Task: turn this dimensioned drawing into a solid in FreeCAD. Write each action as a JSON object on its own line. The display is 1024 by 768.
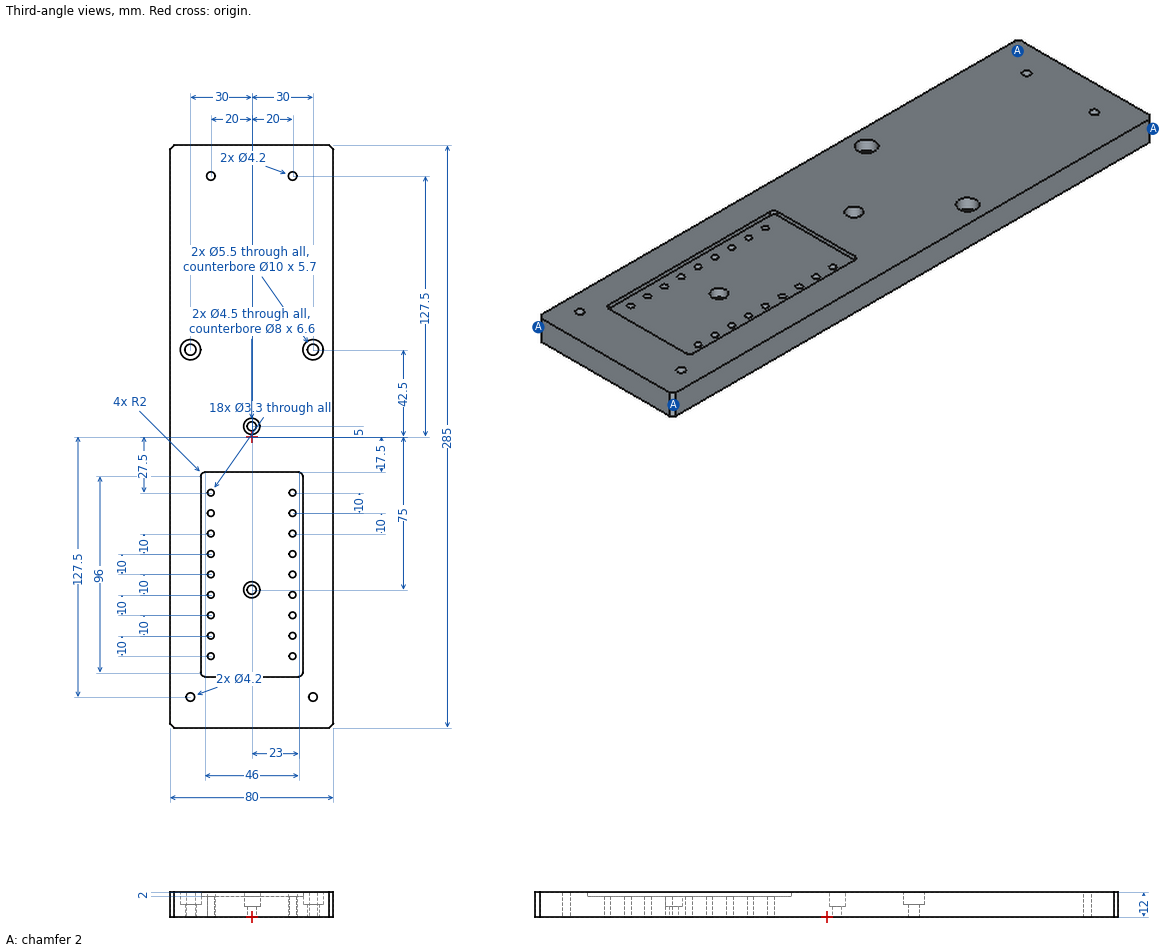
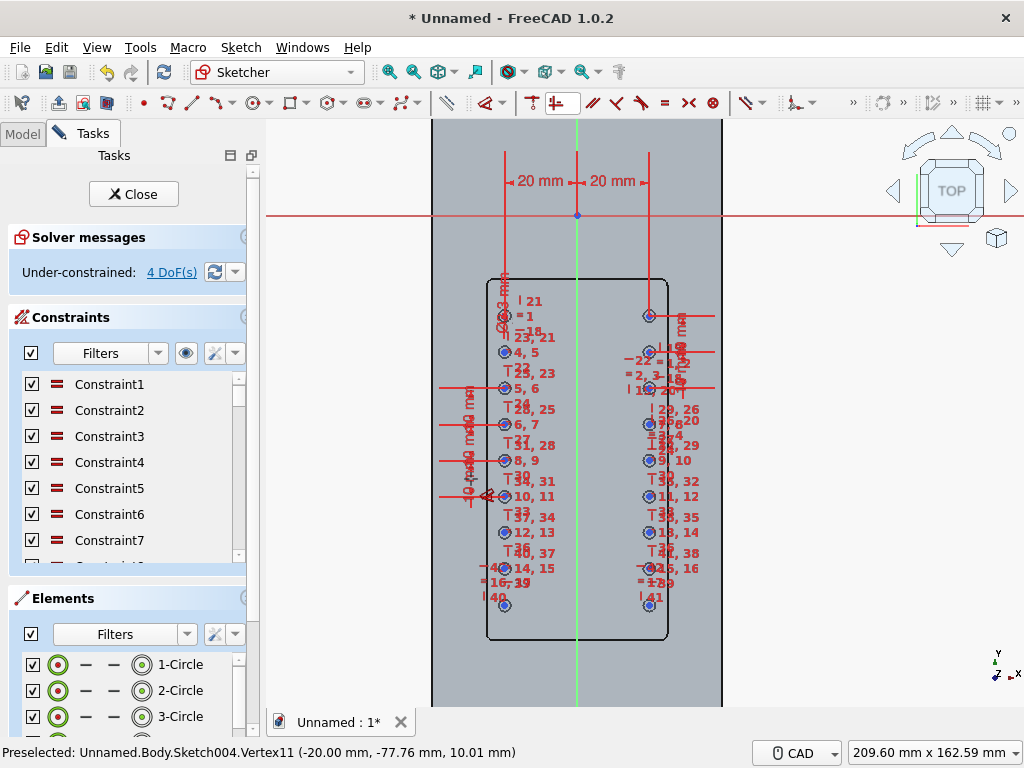
{"action": "left_click", "coordinate": [505, 497]}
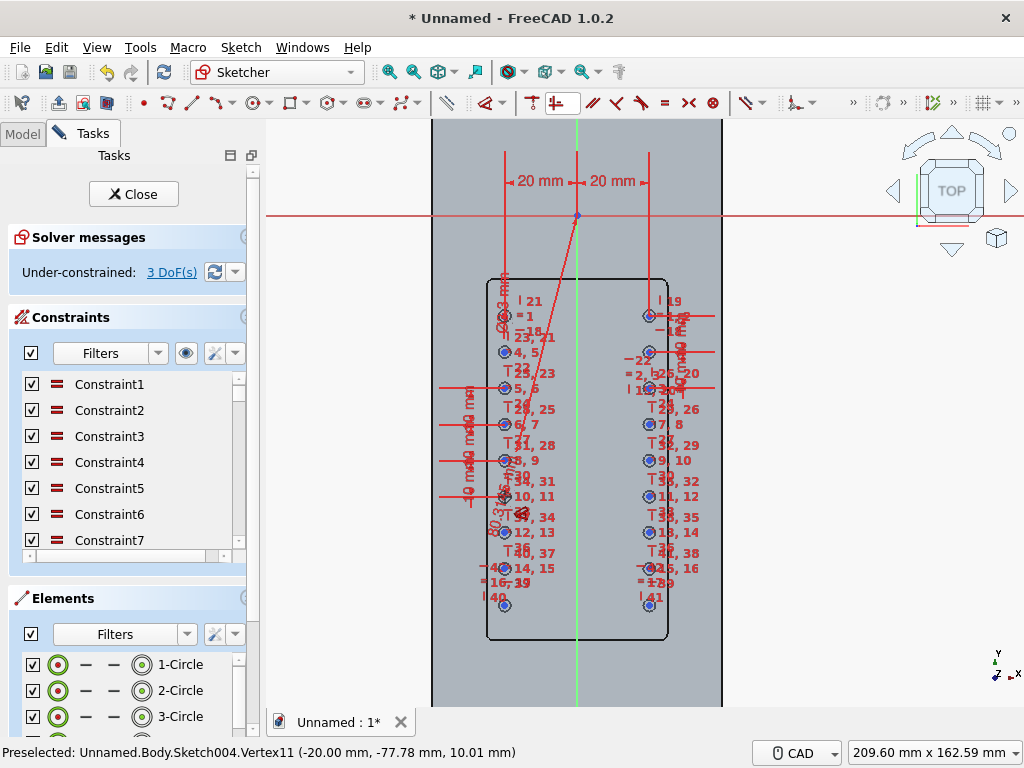
{"action": "left_click", "coordinate": [505, 533]}
{"action": "left_click", "coordinate": [471, 515]}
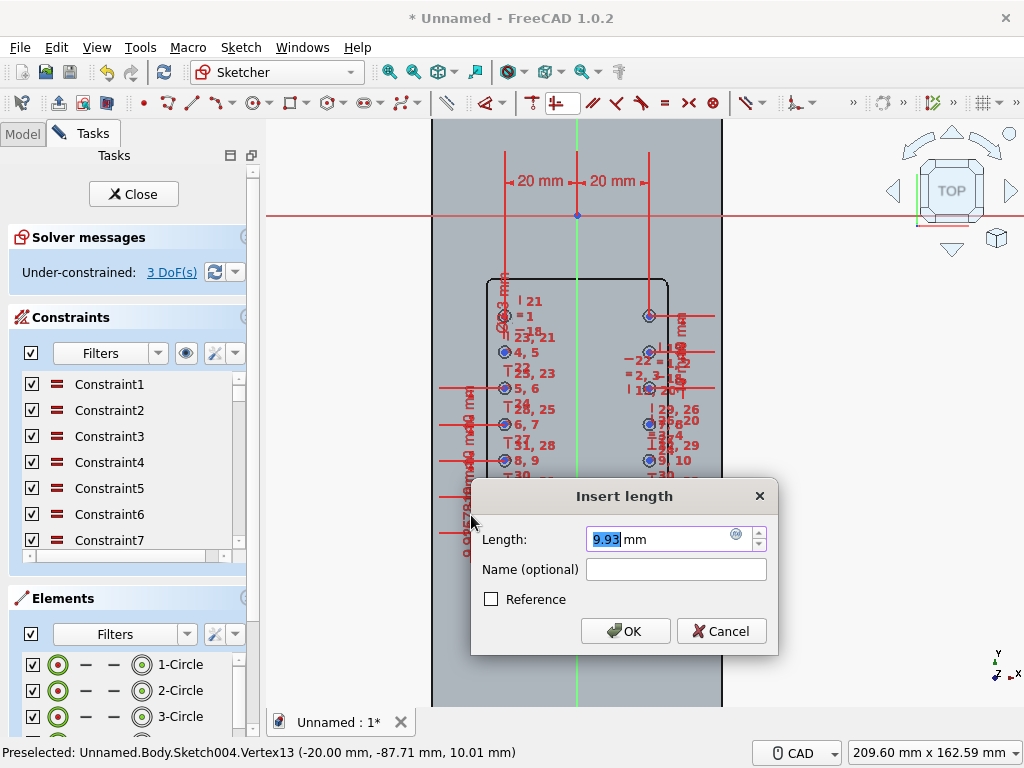
{"action": "type", "text": "10"}
{"action": "key", "text": "Return"}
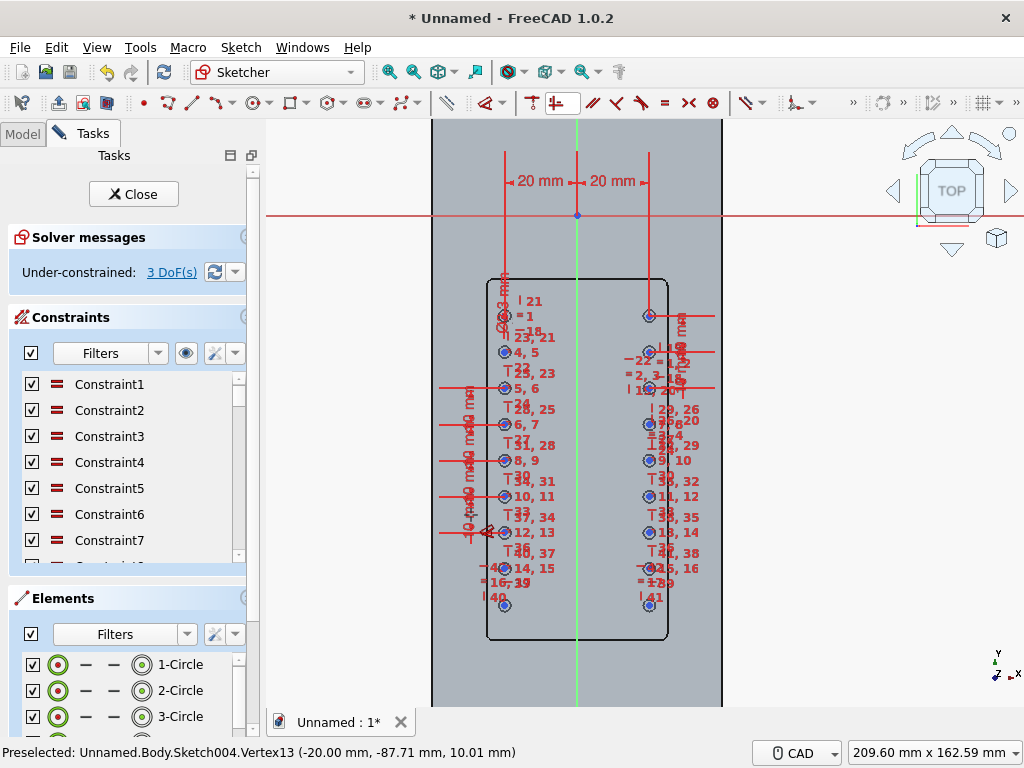
{"action": "left_click", "coordinate": [505, 533]}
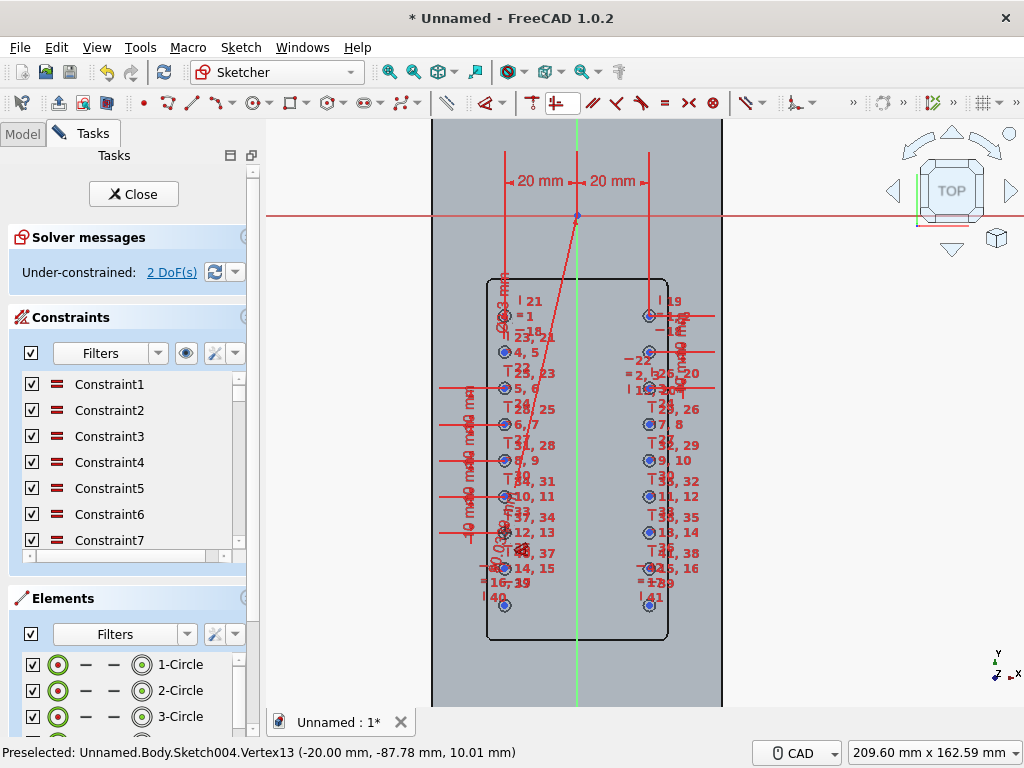
{"action": "left_click", "coordinate": [505, 569]}
{"action": "left_click", "coordinate": [471, 551]}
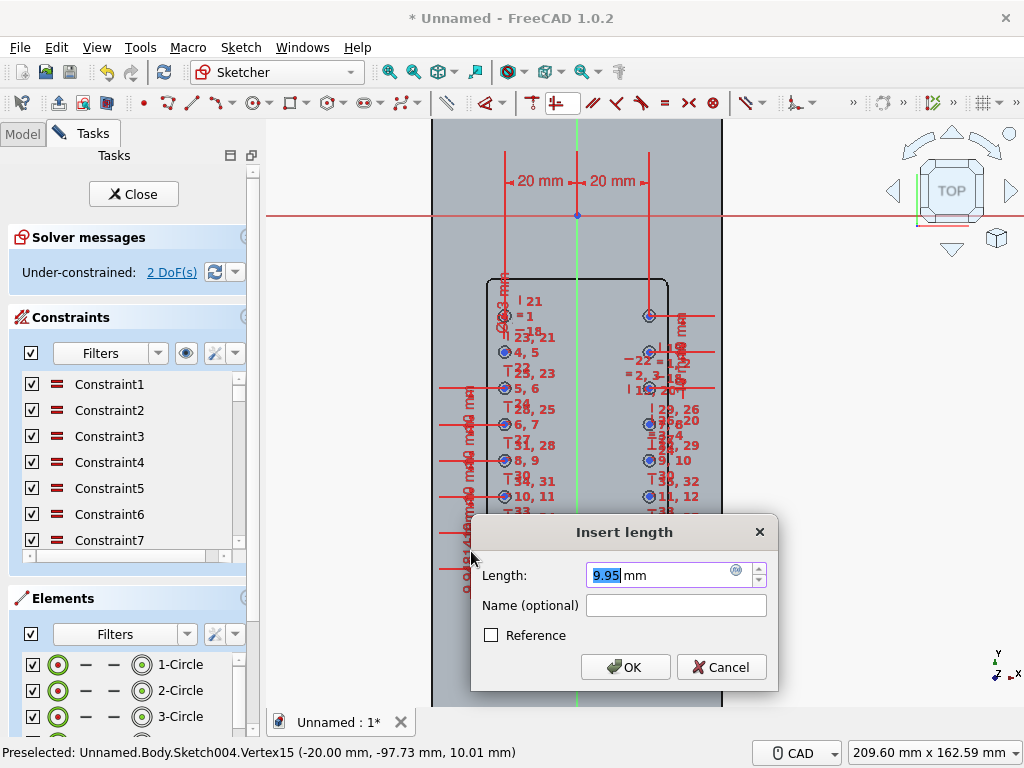
{"action": "type", "text": "10"}
{"action": "key", "text": "Return"}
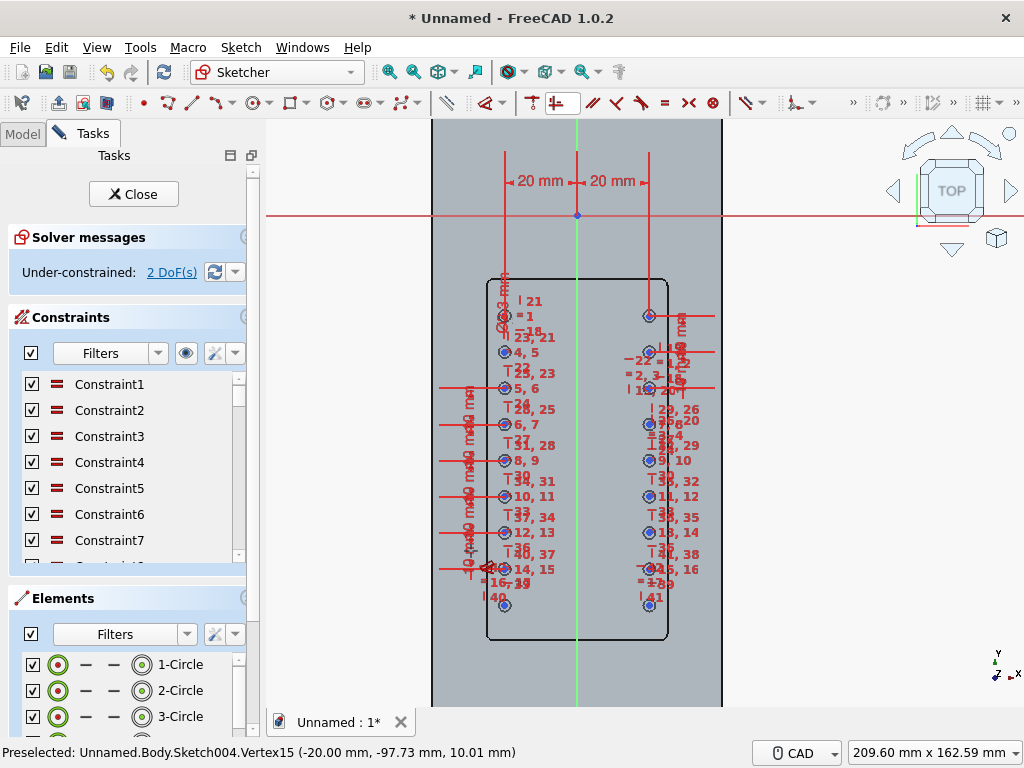
{"action": "left_click", "coordinate": [505, 569]}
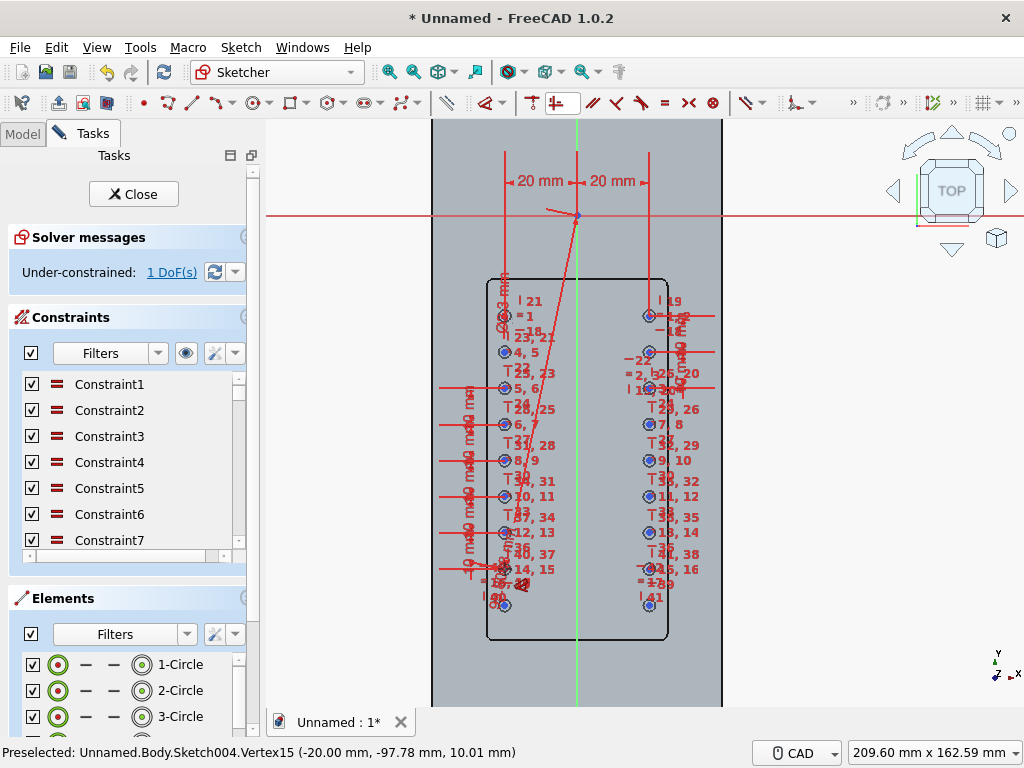
{"action": "left_click", "coordinate": [505, 606]}
{"action": "left_click", "coordinate": [471, 587]}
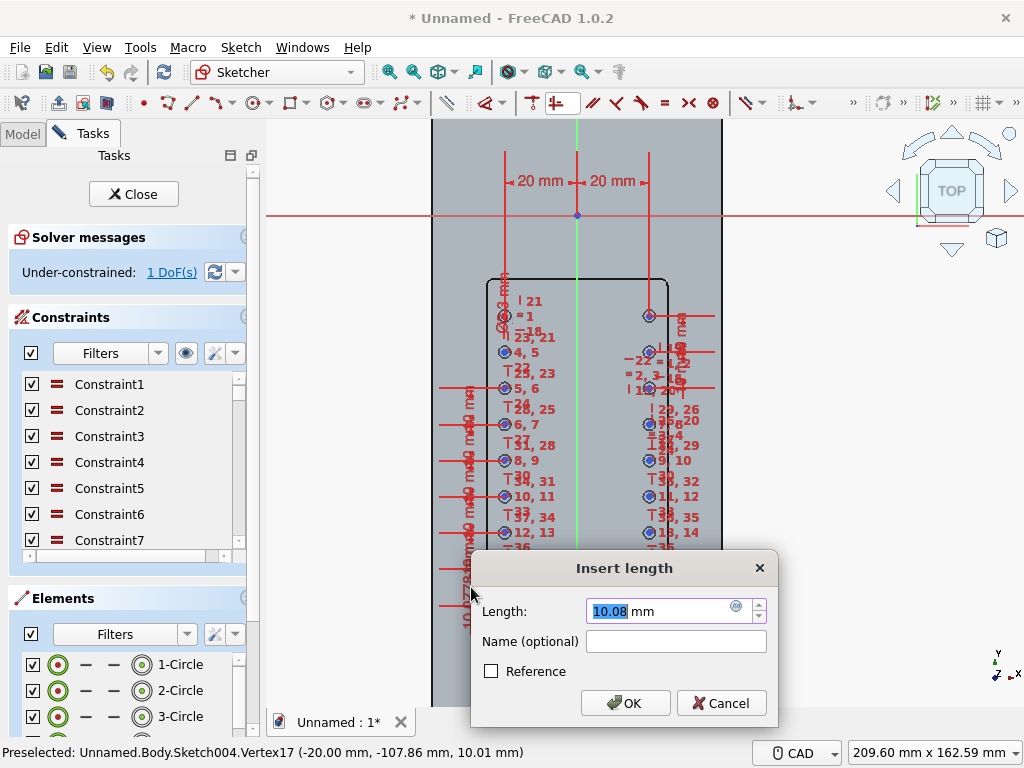
{"action": "type", "text": "10"}
{"action": "key", "text": "Return"}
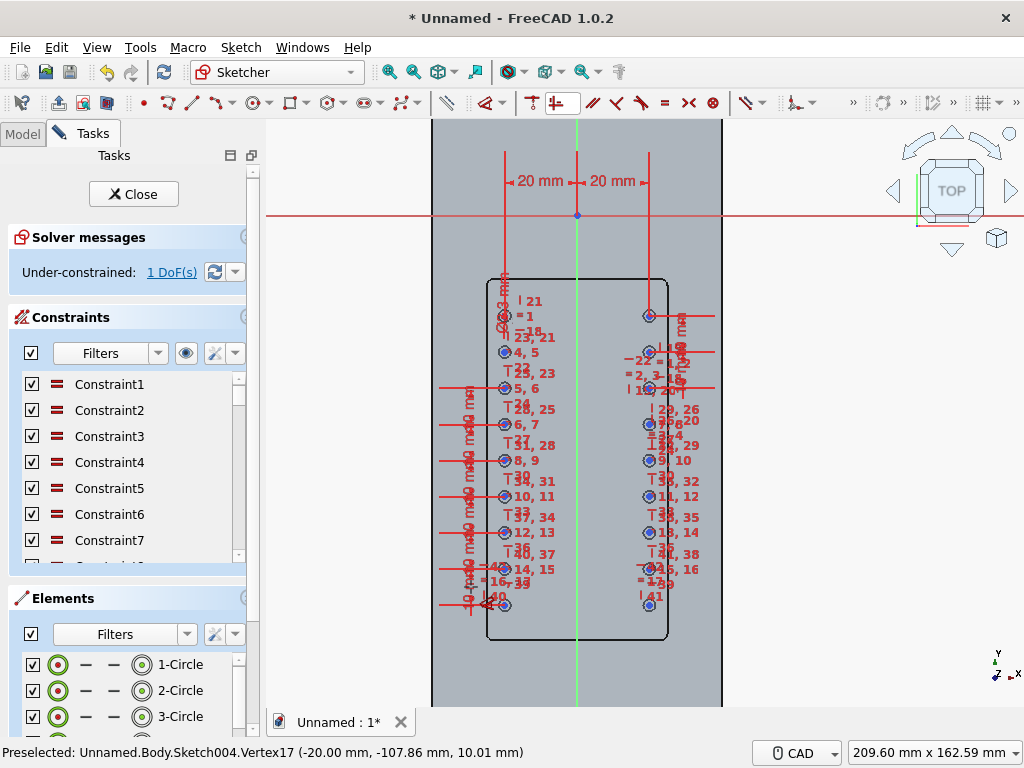
{"action": "left_click", "coordinate": [505, 316]}
{"action": "left_click", "coordinate": [471, 266]}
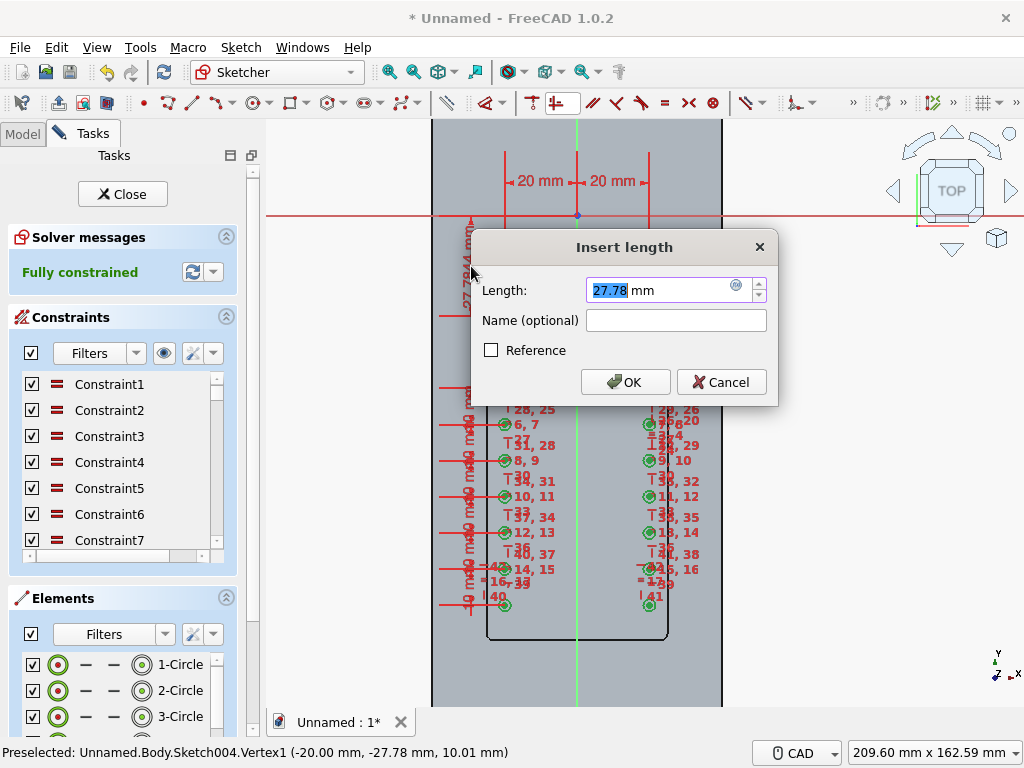
{"action": "type", "text": "27.5"}
{"action": "key", "text": "Return"}
{"action": "key", "text": "Escape"}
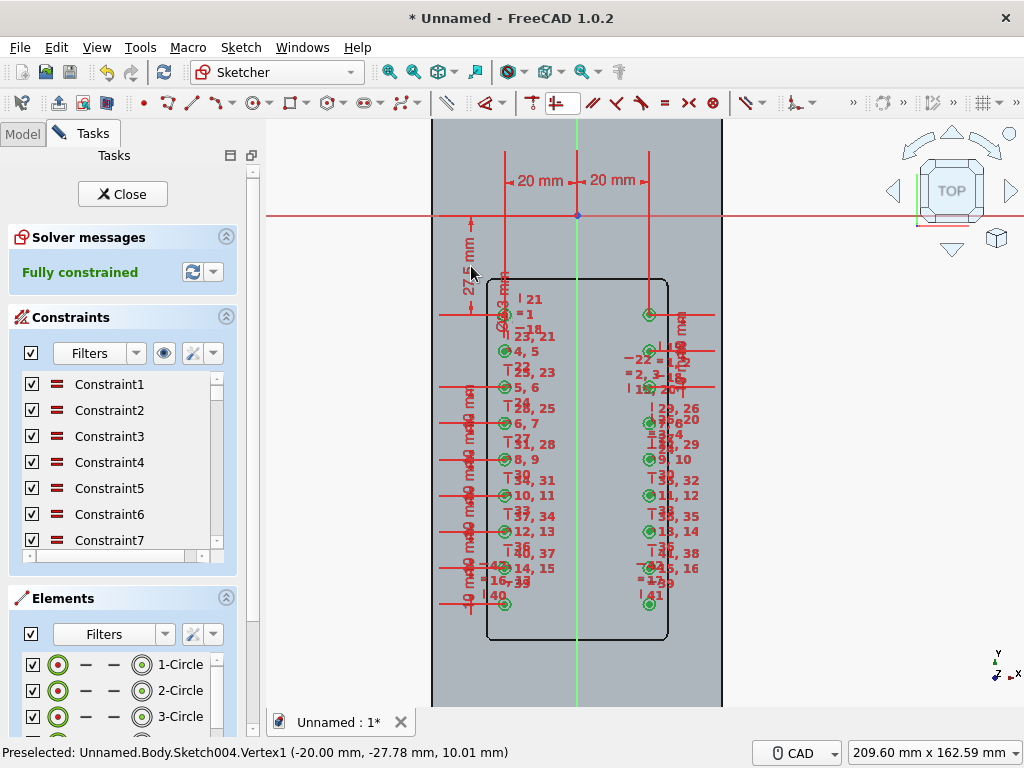
{"action": "left_click", "coordinate": [123, 194]}